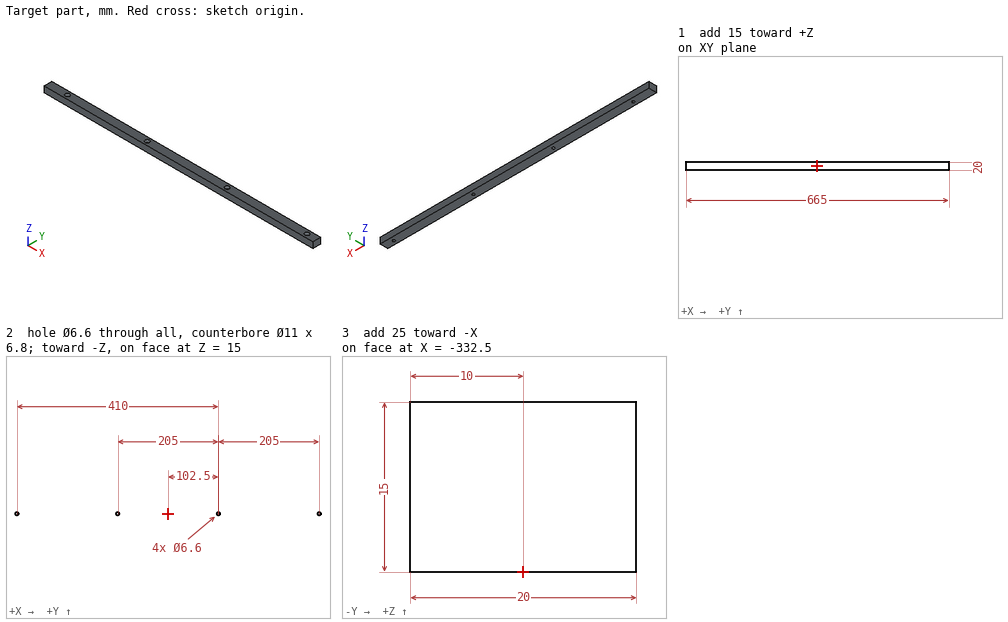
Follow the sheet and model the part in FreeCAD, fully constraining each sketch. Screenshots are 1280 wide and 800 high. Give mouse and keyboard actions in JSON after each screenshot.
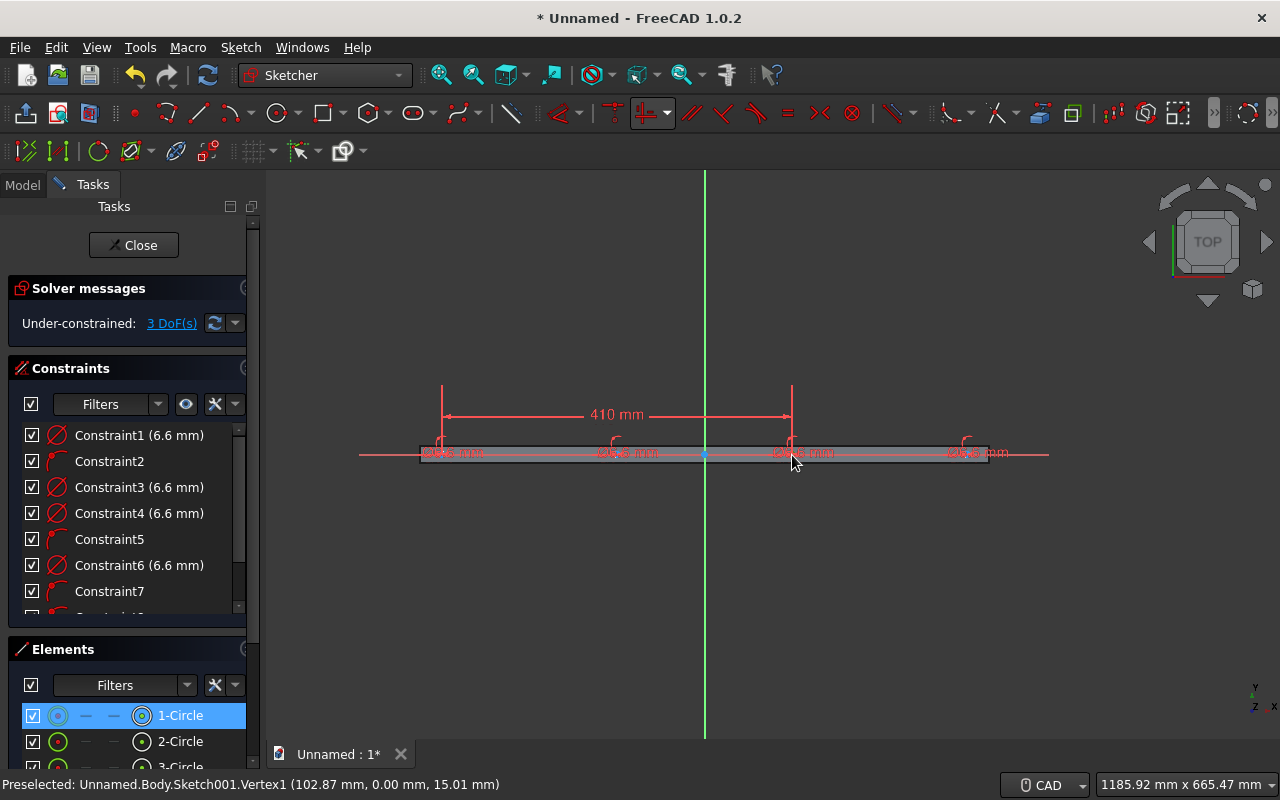
{"action": "left_click", "coordinate": [967, 455]}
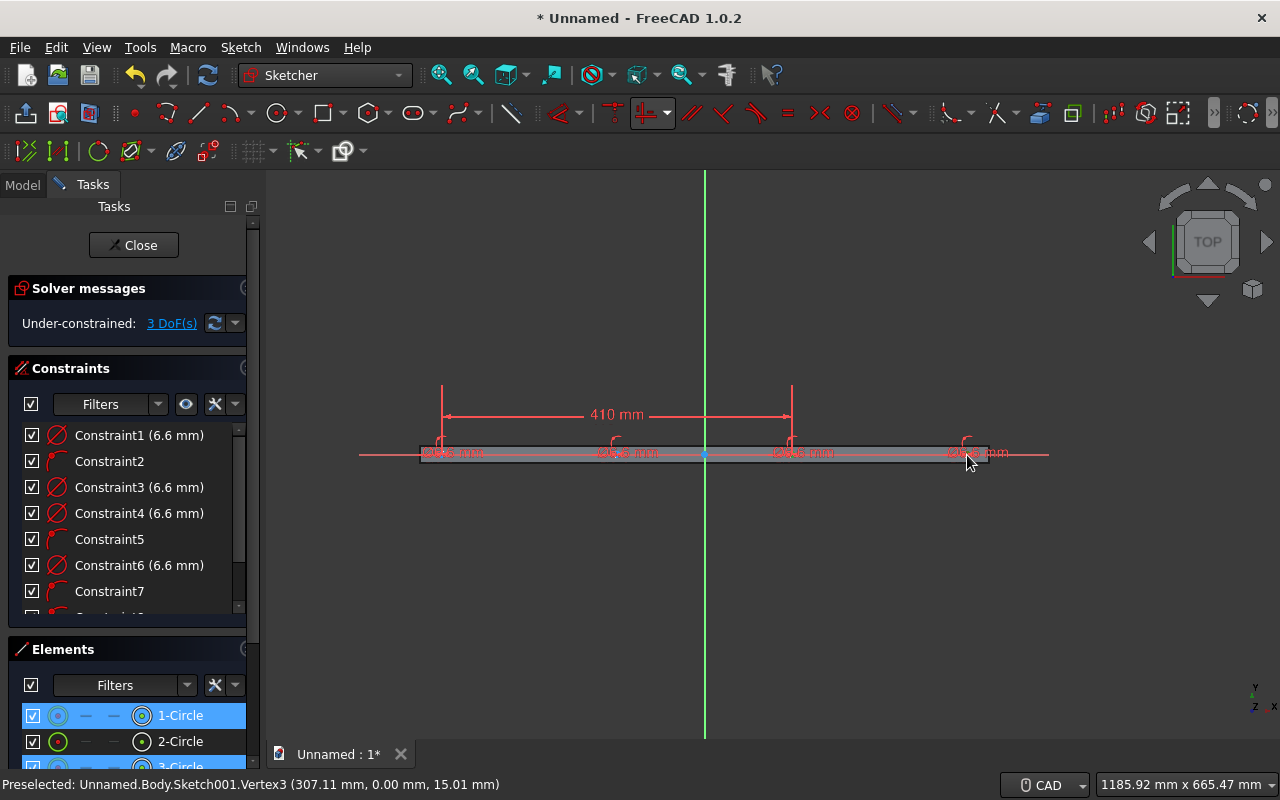
{"action": "key", "text": "l"}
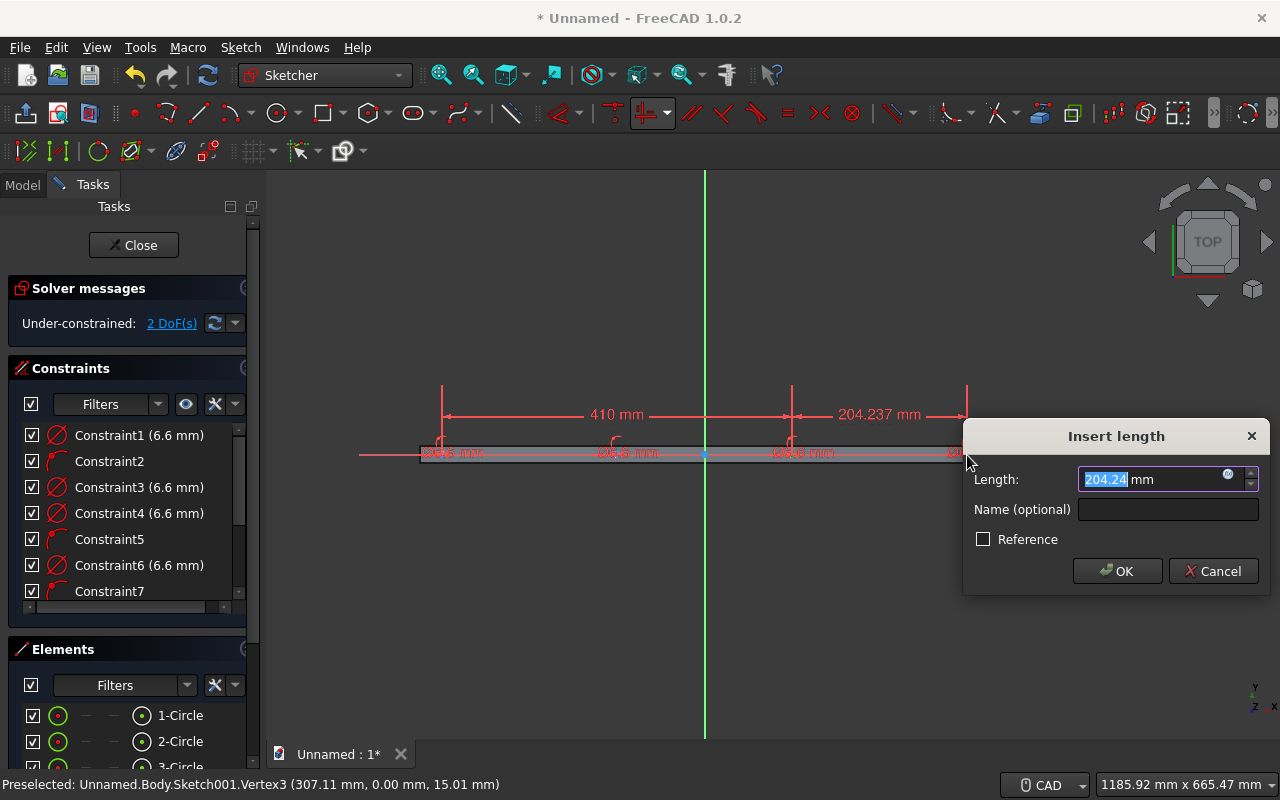
{"action": "type", "text": "205"}
{"action": "key", "text": "Return"}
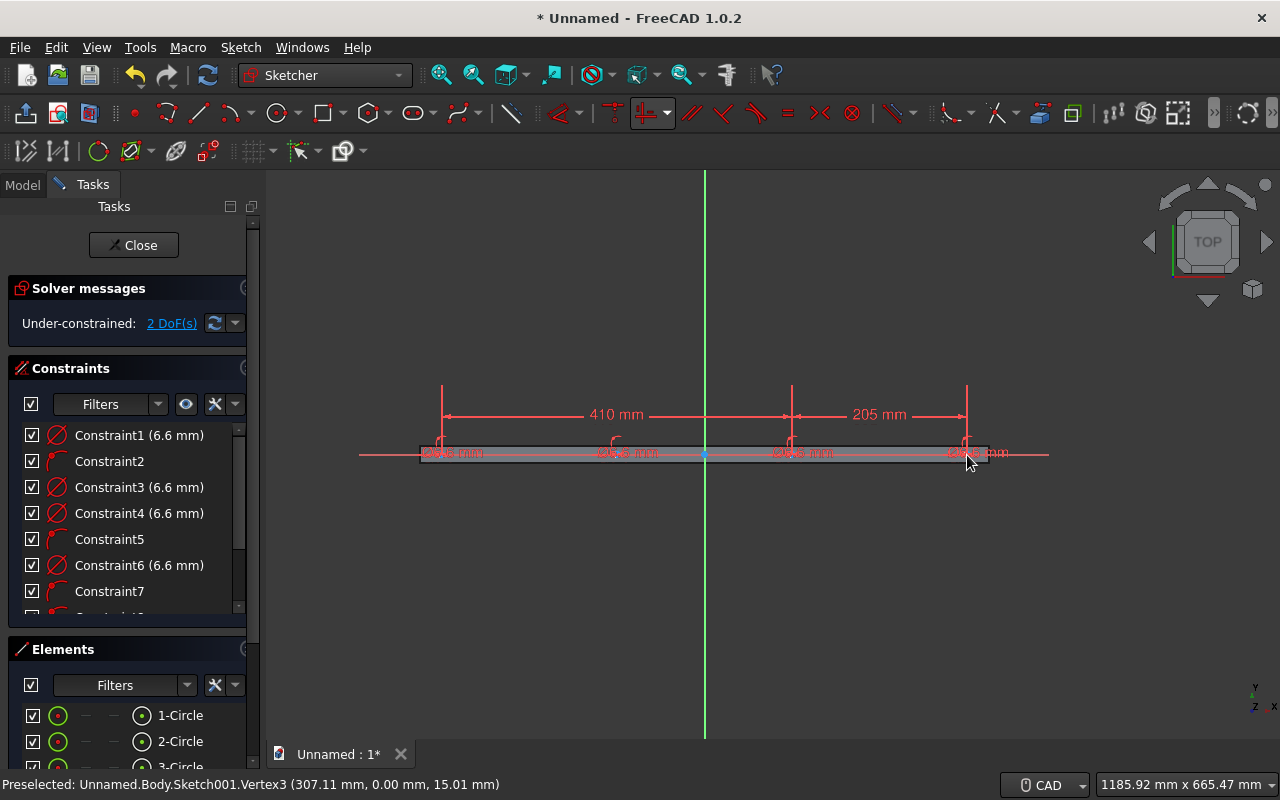
{"action": "left_click", "coordinate": [792, 455]}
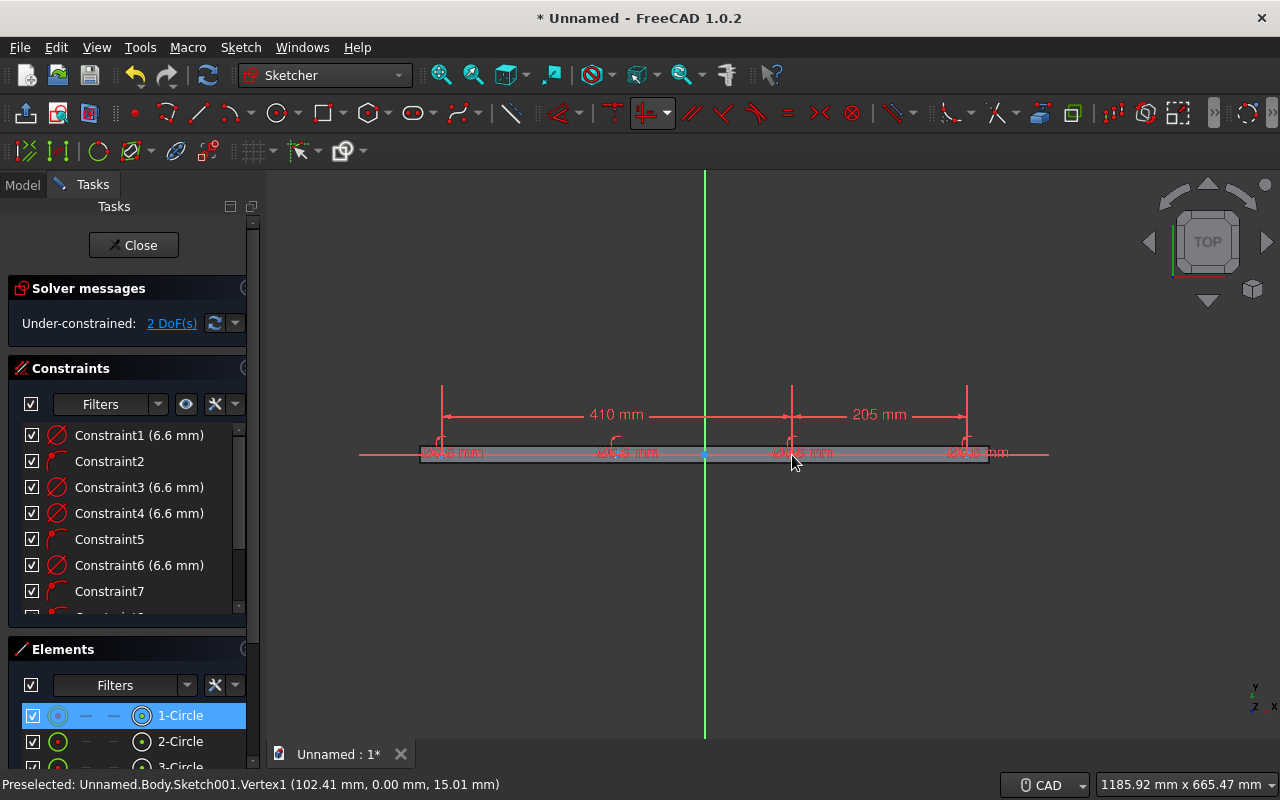
{"action": "left_click", "coordinate": [617, 455]}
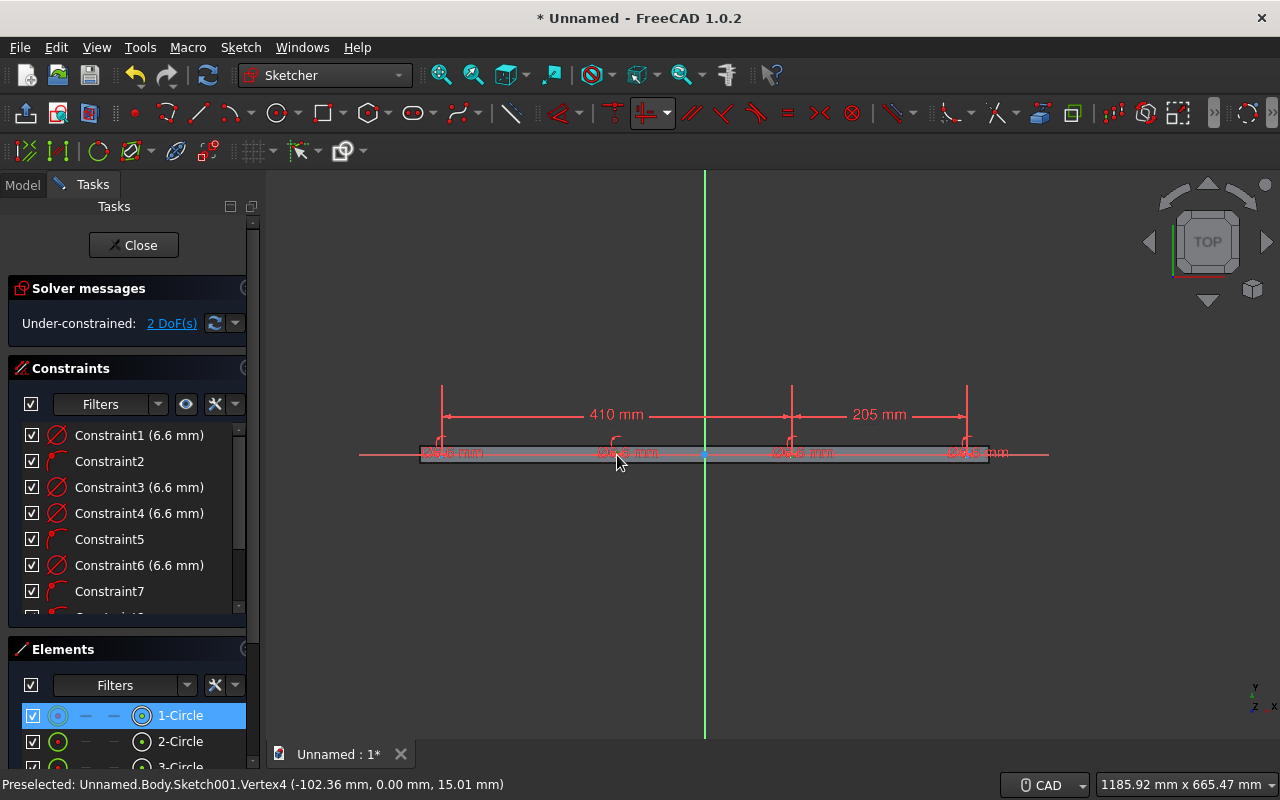
{"action": "key", "text": "l"}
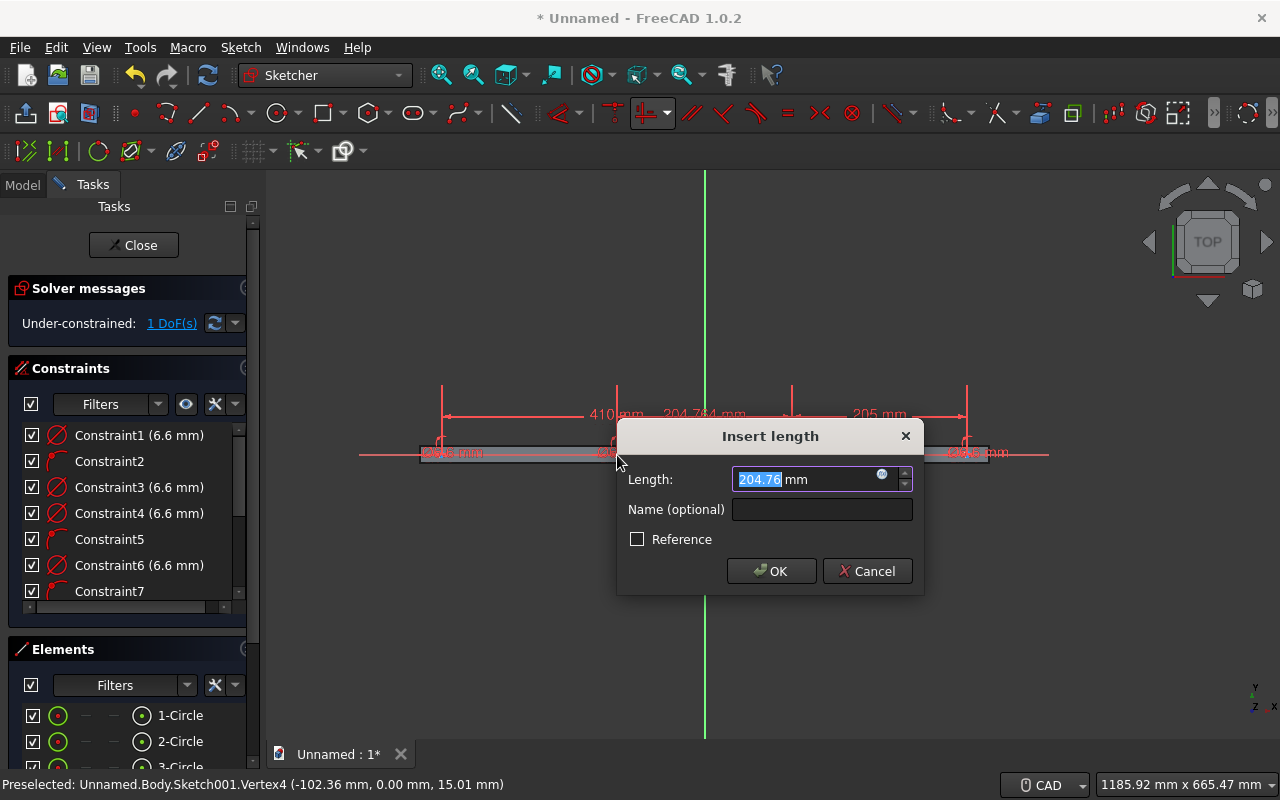
{"action": "type", "text": "205"}
{"action": "key", "text": "Return"}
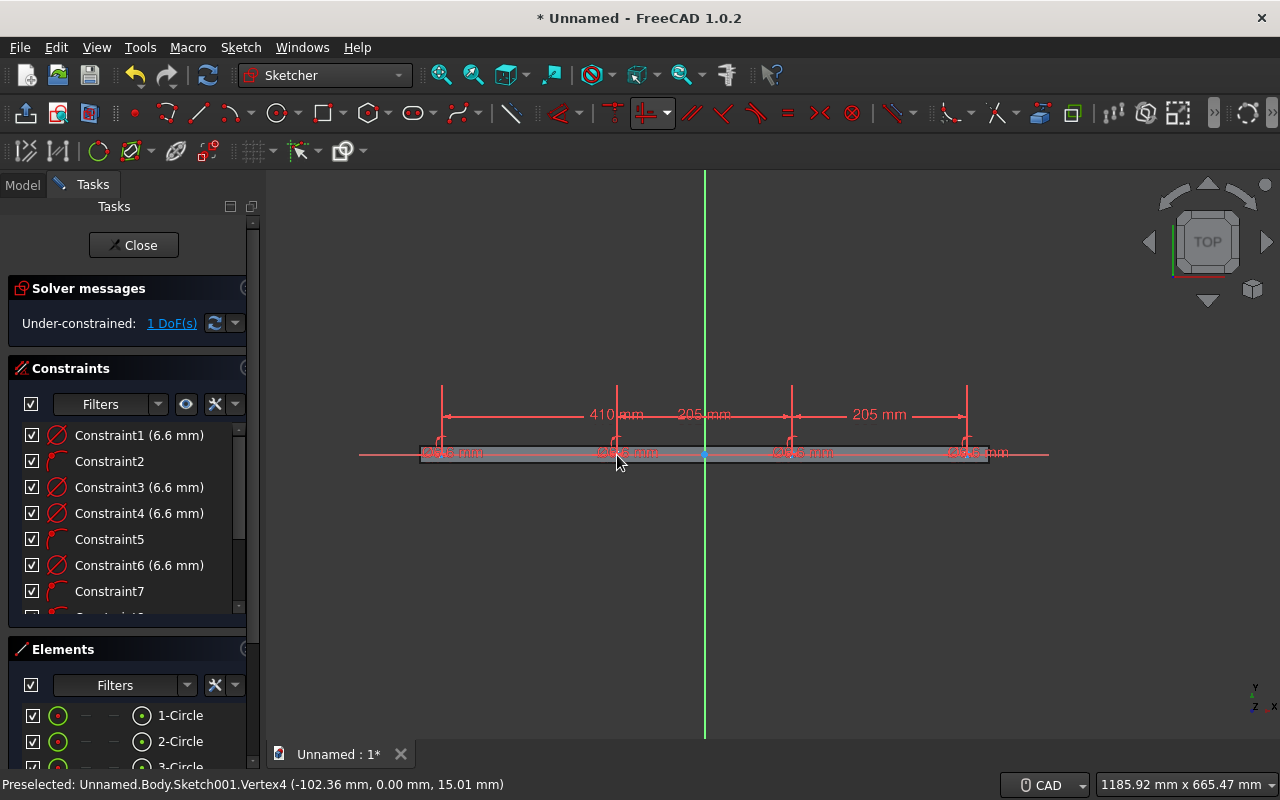
{"action": "left_click", "coordinate": [792, 455]}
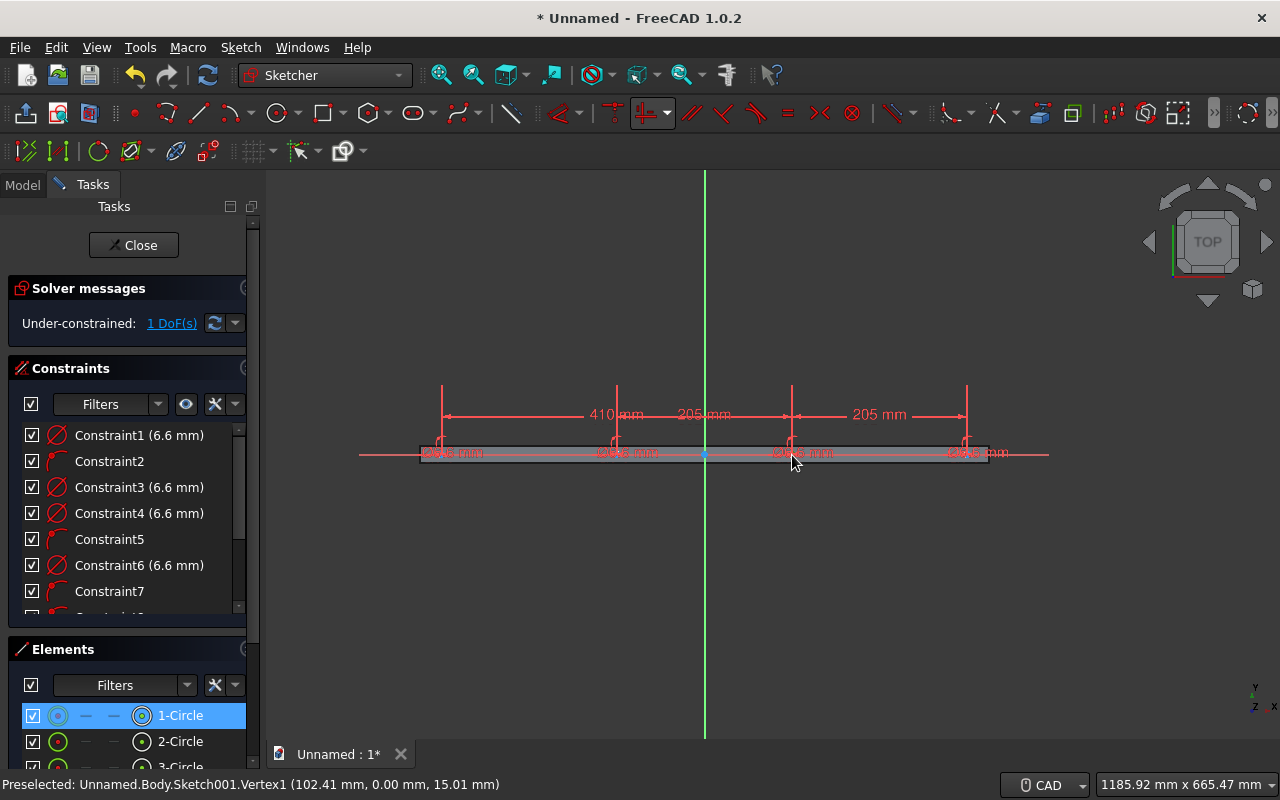
{"action": "key", "text": "l"}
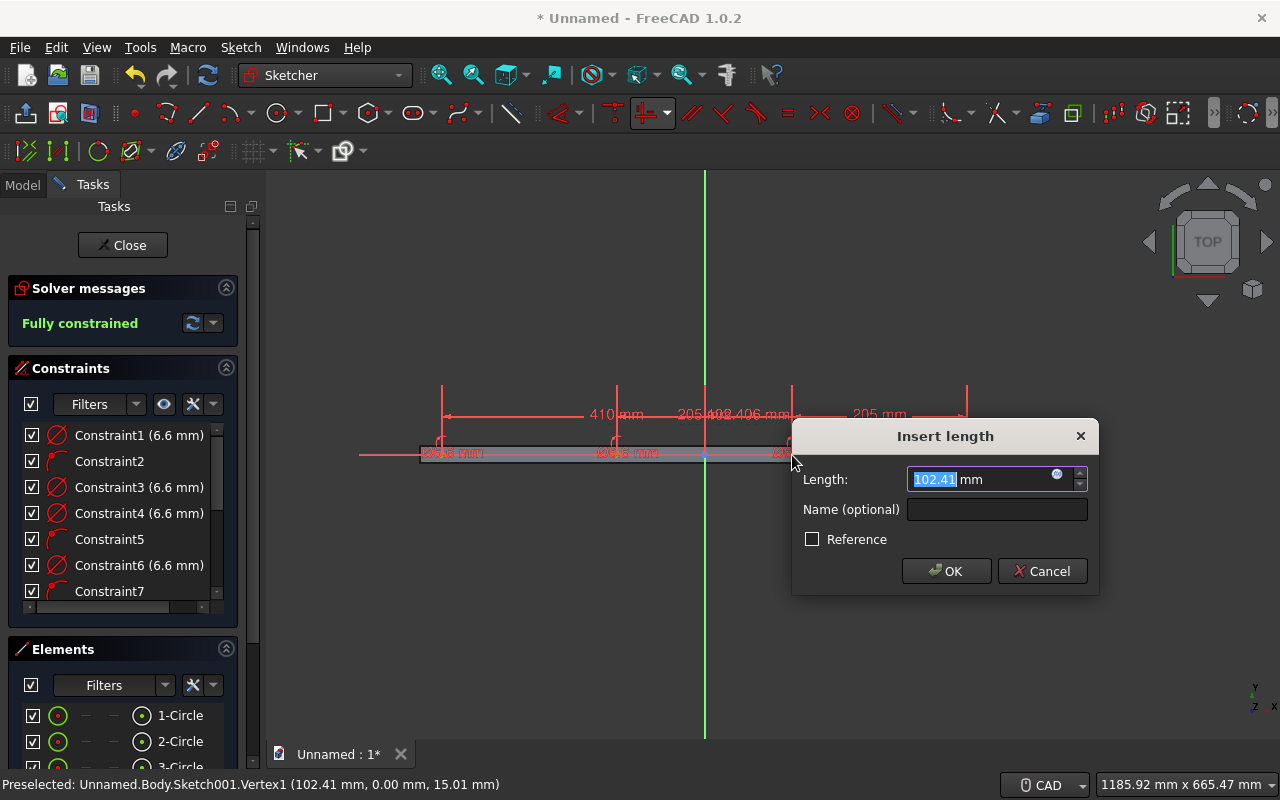
{"action": "type", "text": "102.5"}
{"action": "key", "text": "Return"}